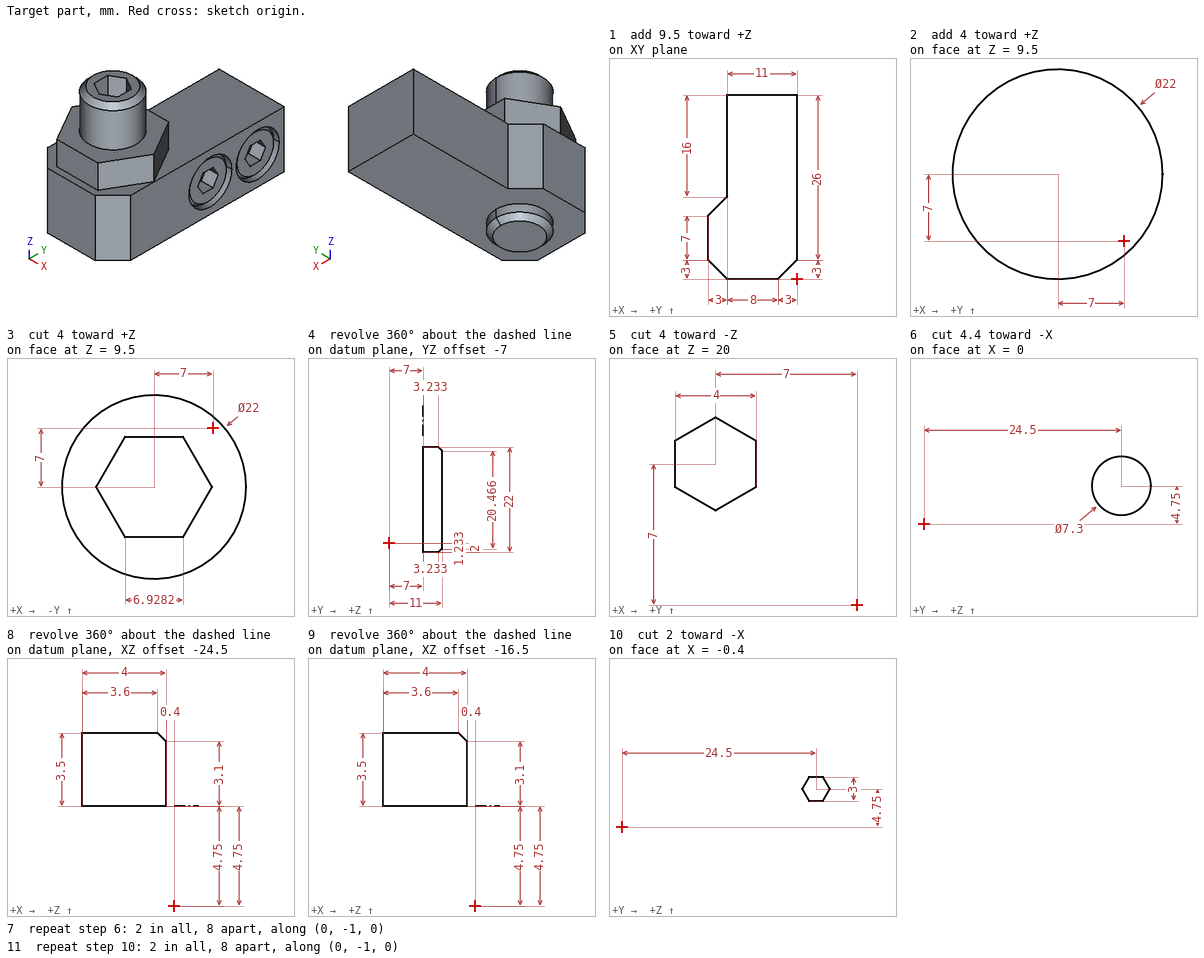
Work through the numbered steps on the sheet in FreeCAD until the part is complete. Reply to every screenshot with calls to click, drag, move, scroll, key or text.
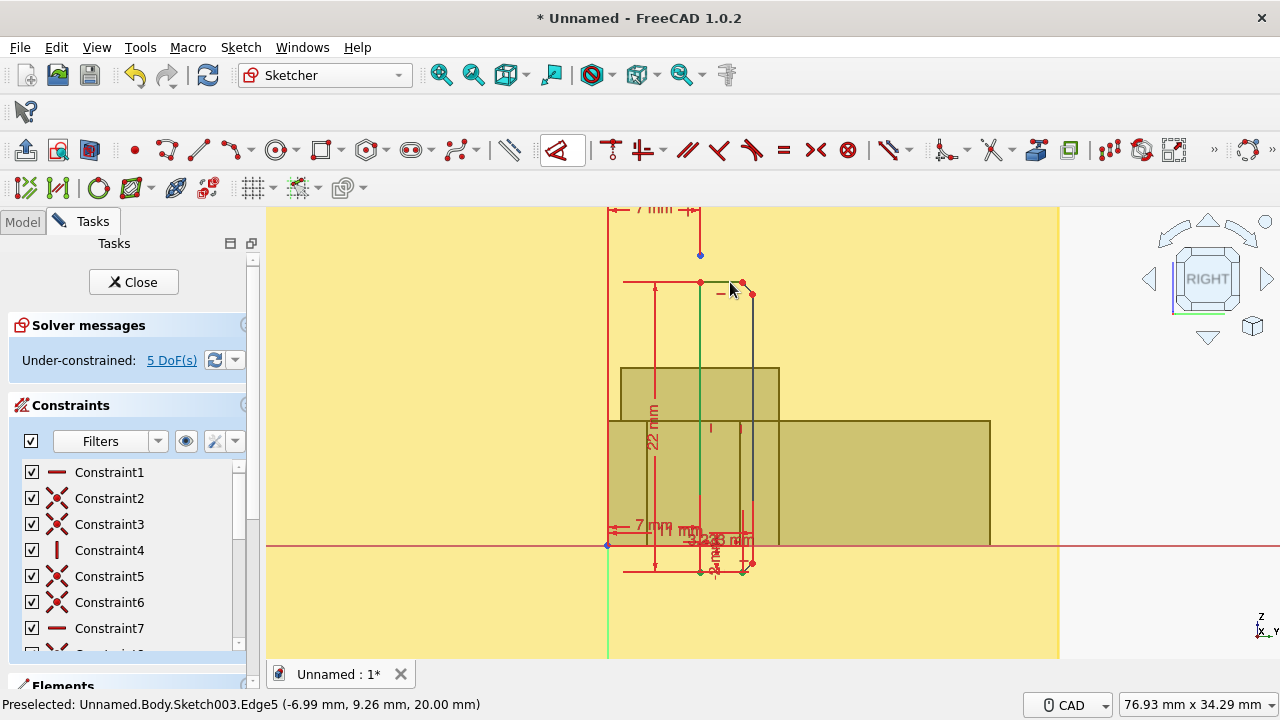
key(l)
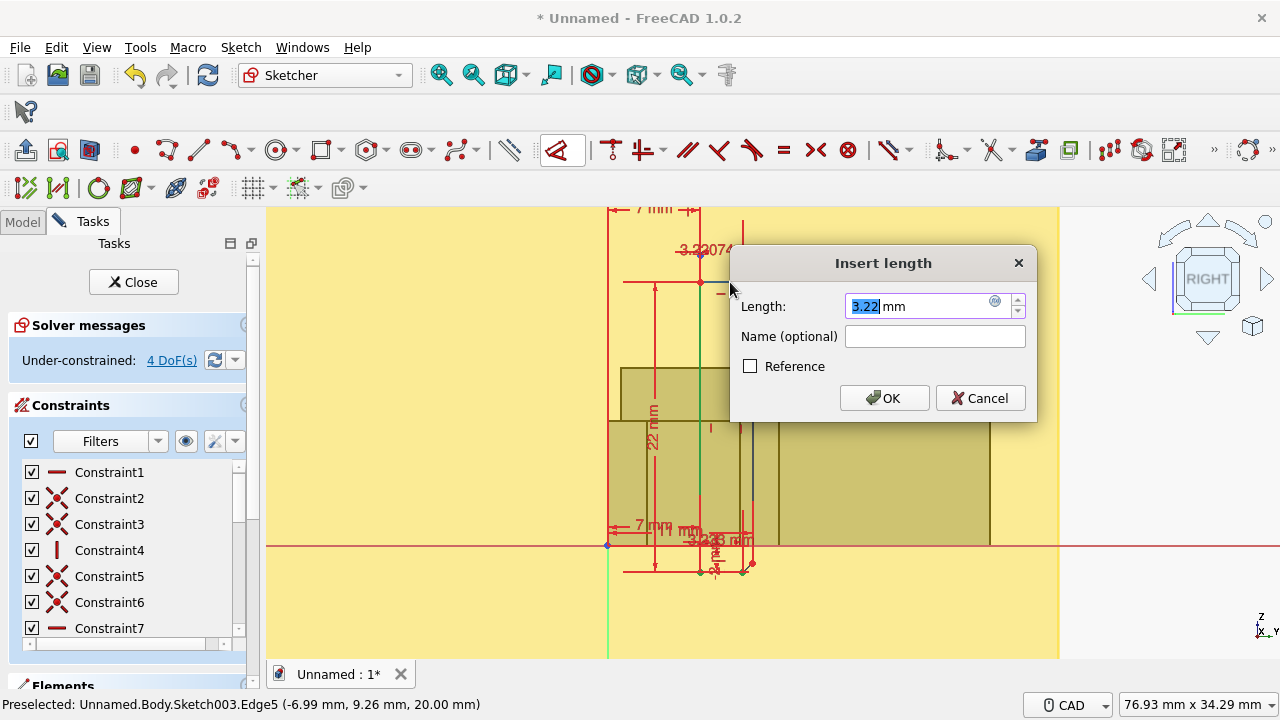
text(3.233)
key(Return)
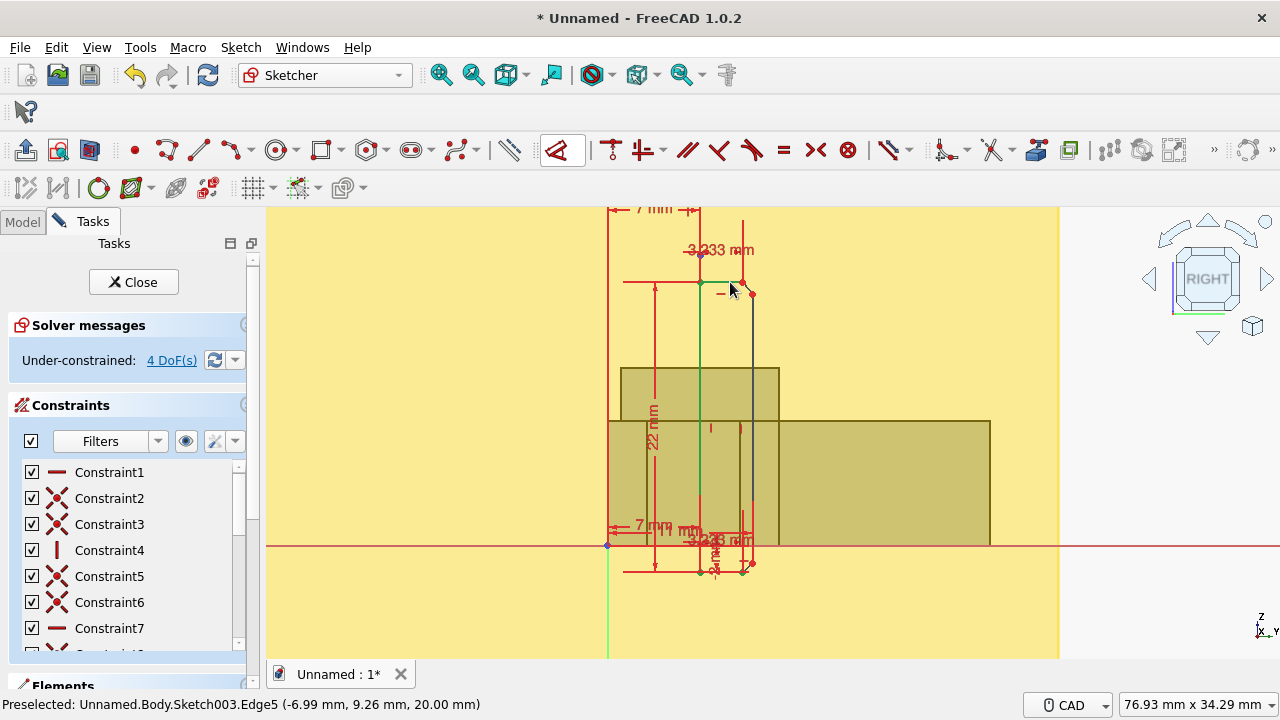
click(753, 482)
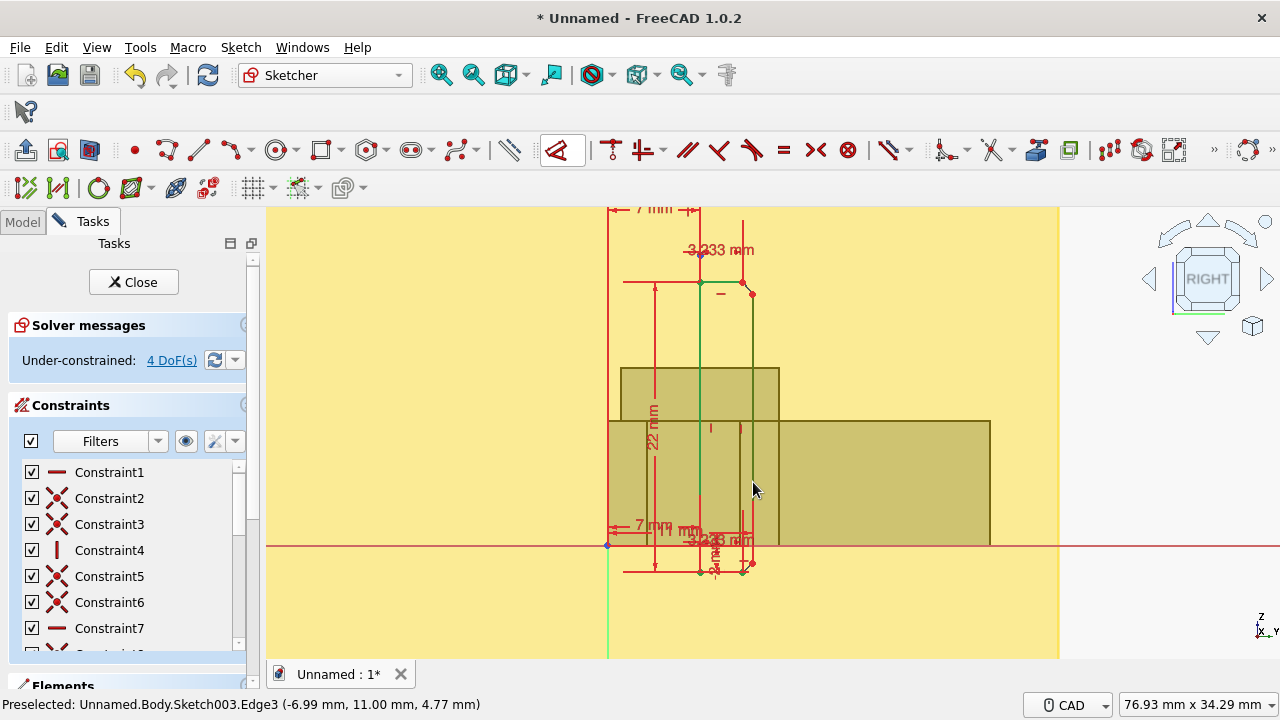
key(i)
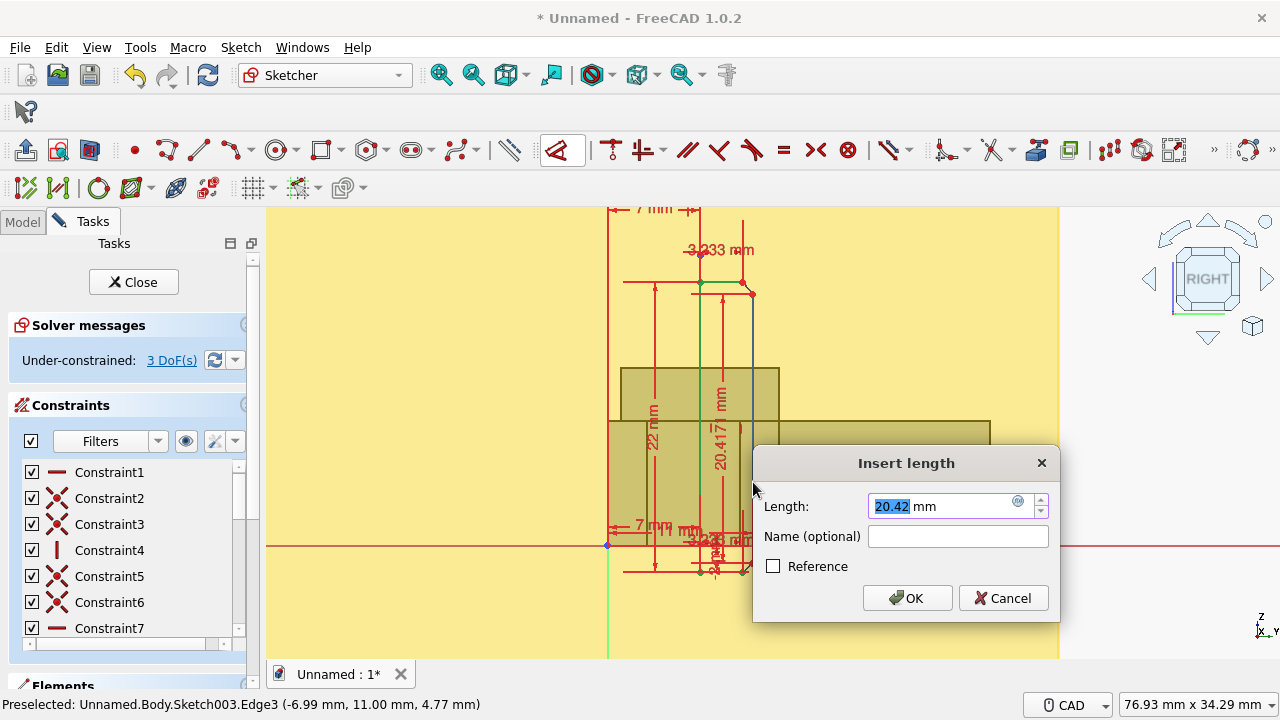
text(20.466)
key(Return)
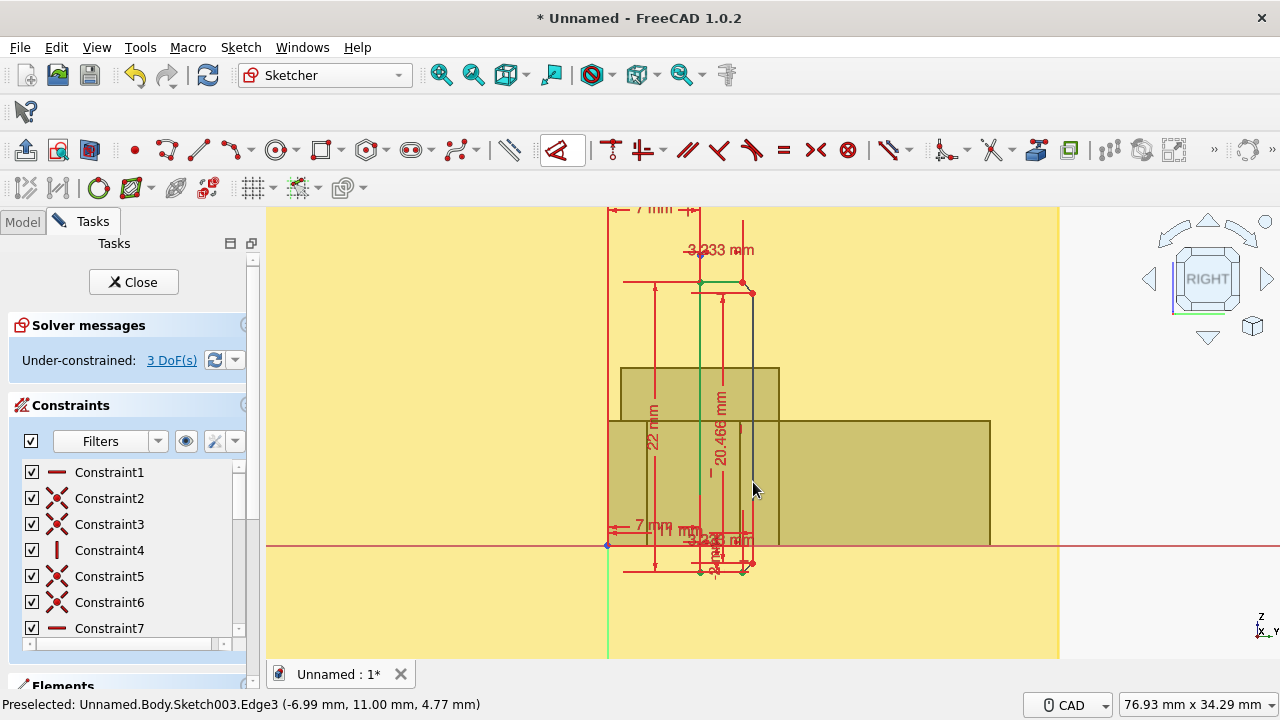
scroll(753, 563, up, 5)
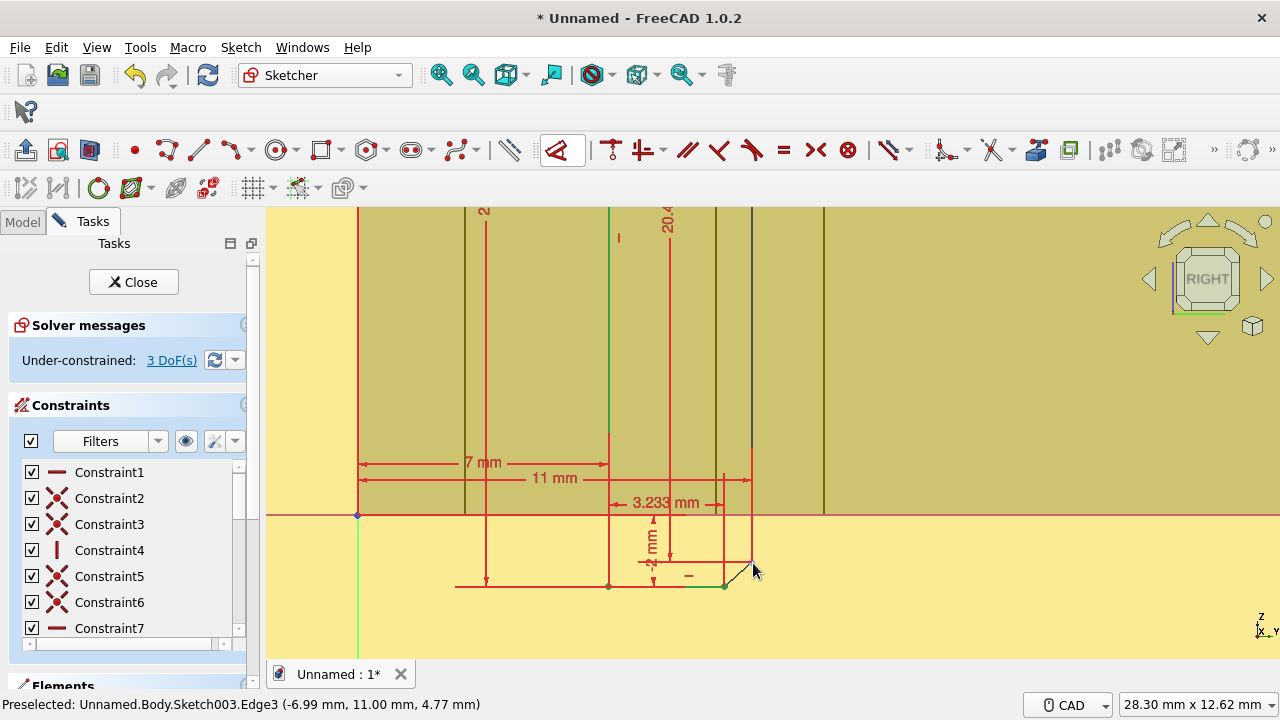
click(752, 562)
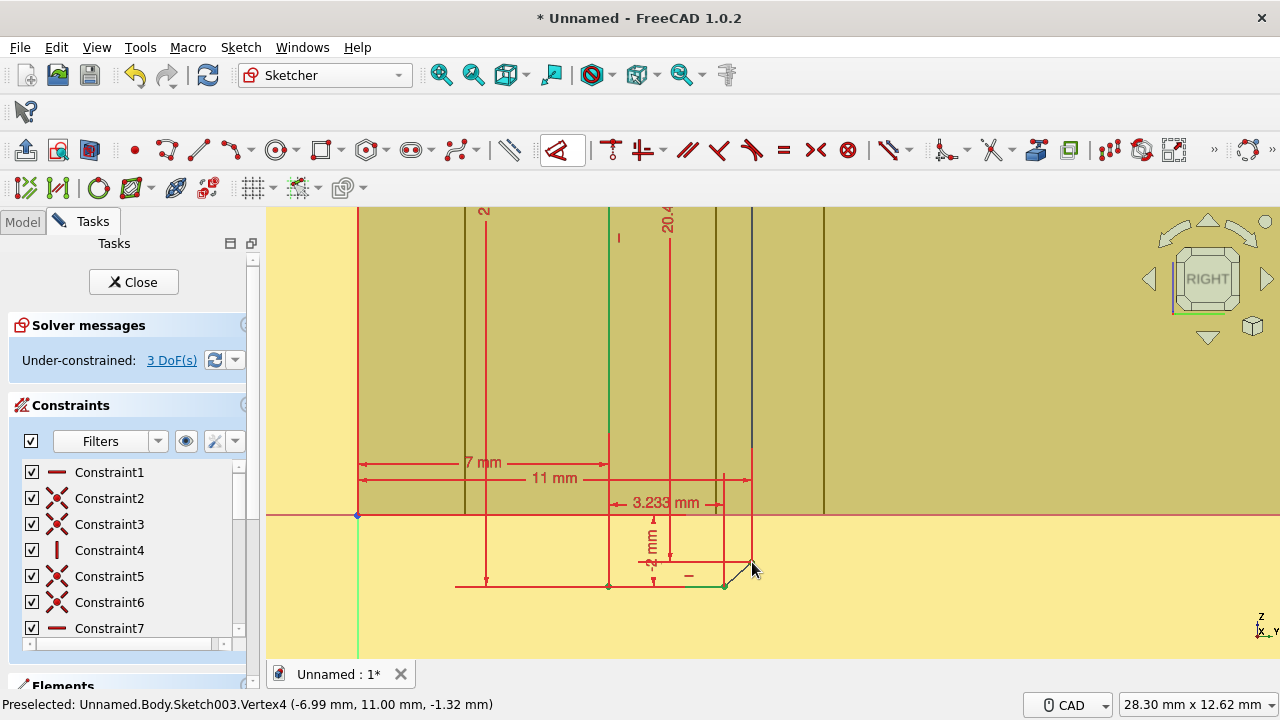
click(580, 150)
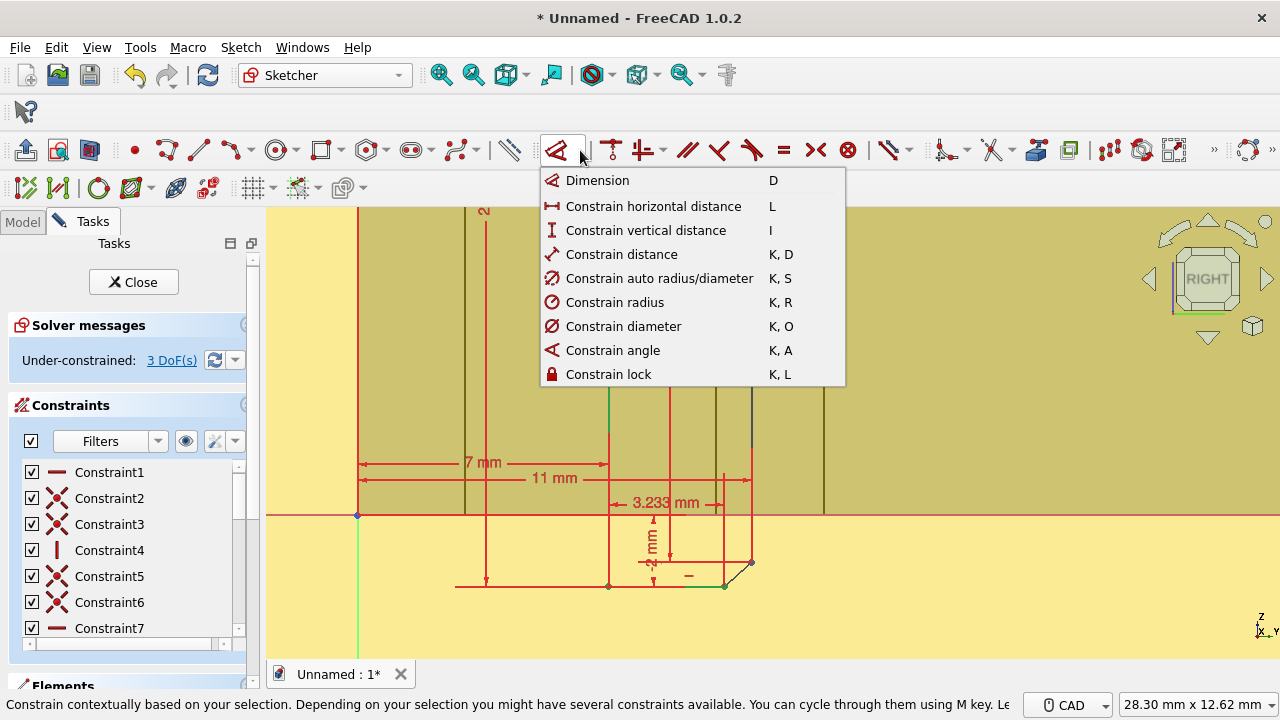
click(693, 230)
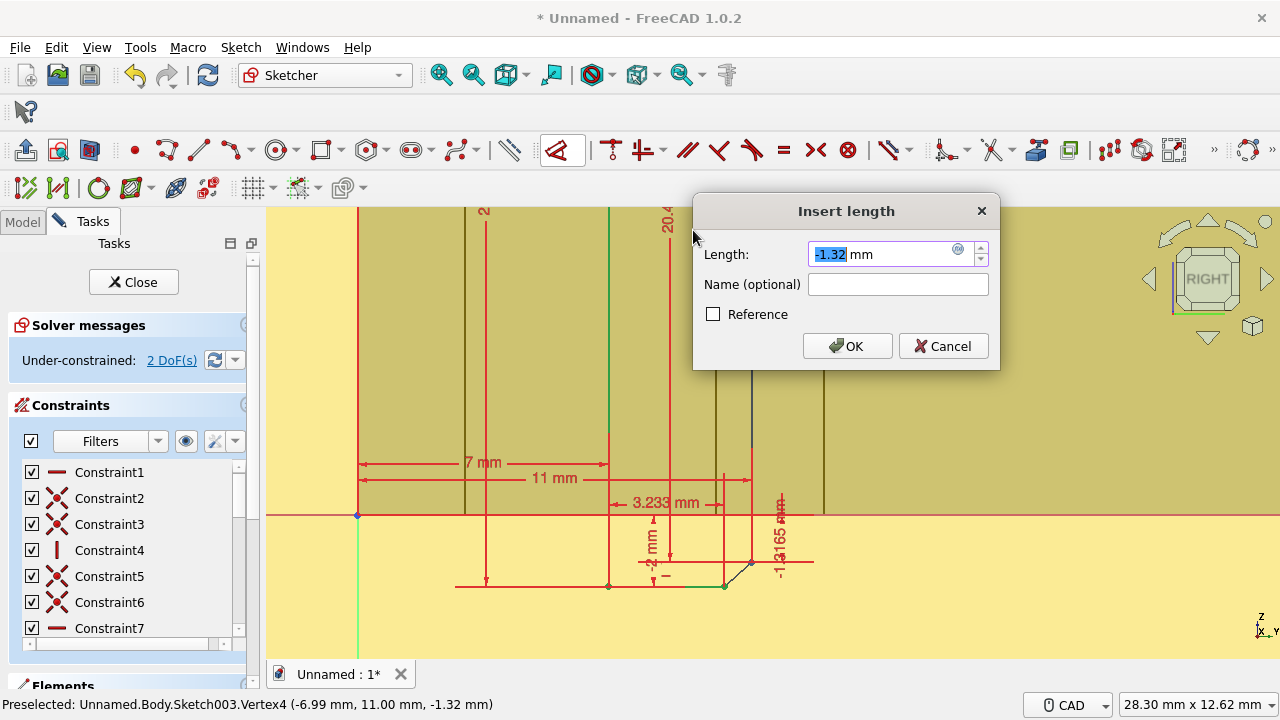
text(-1.233)
key(Return)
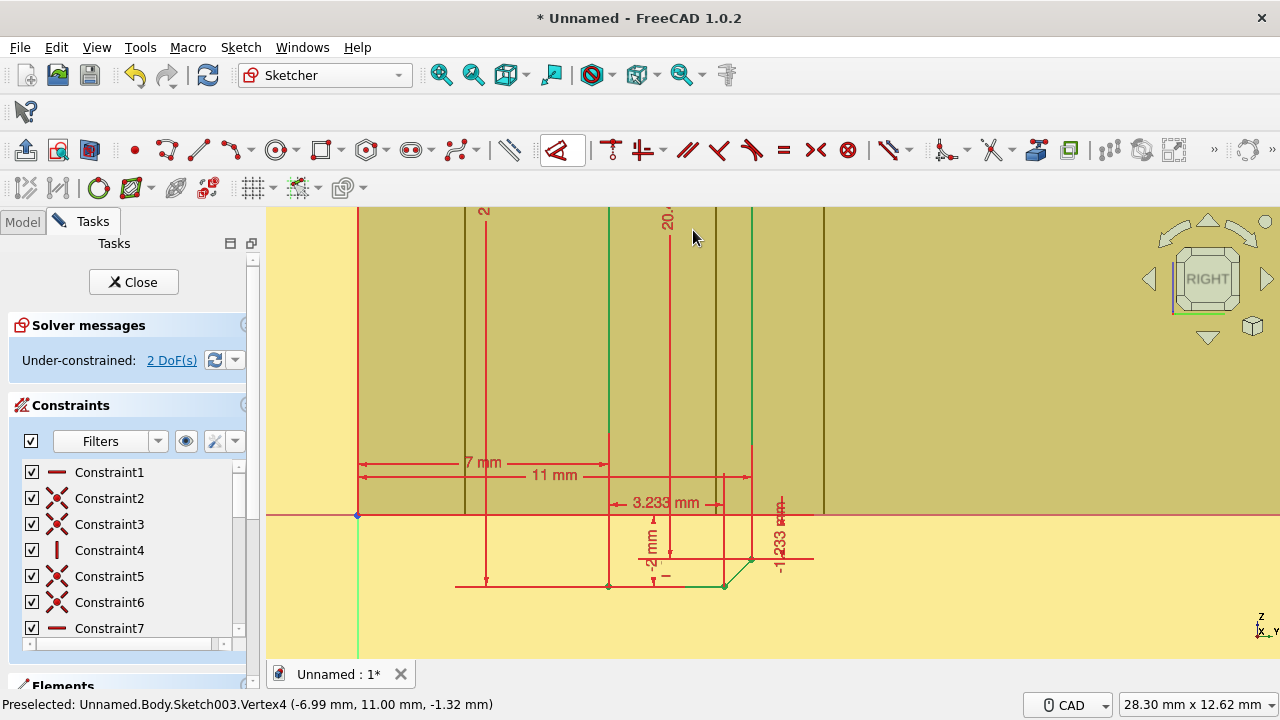
click(134, 282)